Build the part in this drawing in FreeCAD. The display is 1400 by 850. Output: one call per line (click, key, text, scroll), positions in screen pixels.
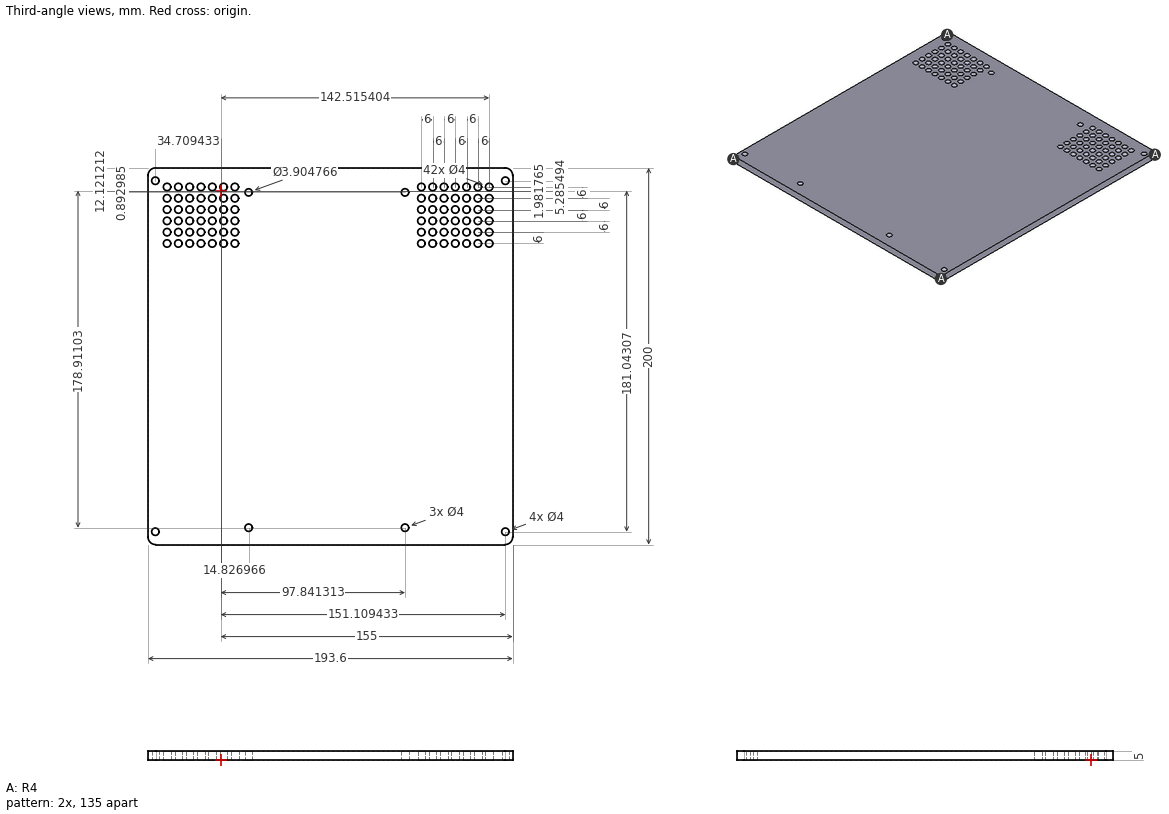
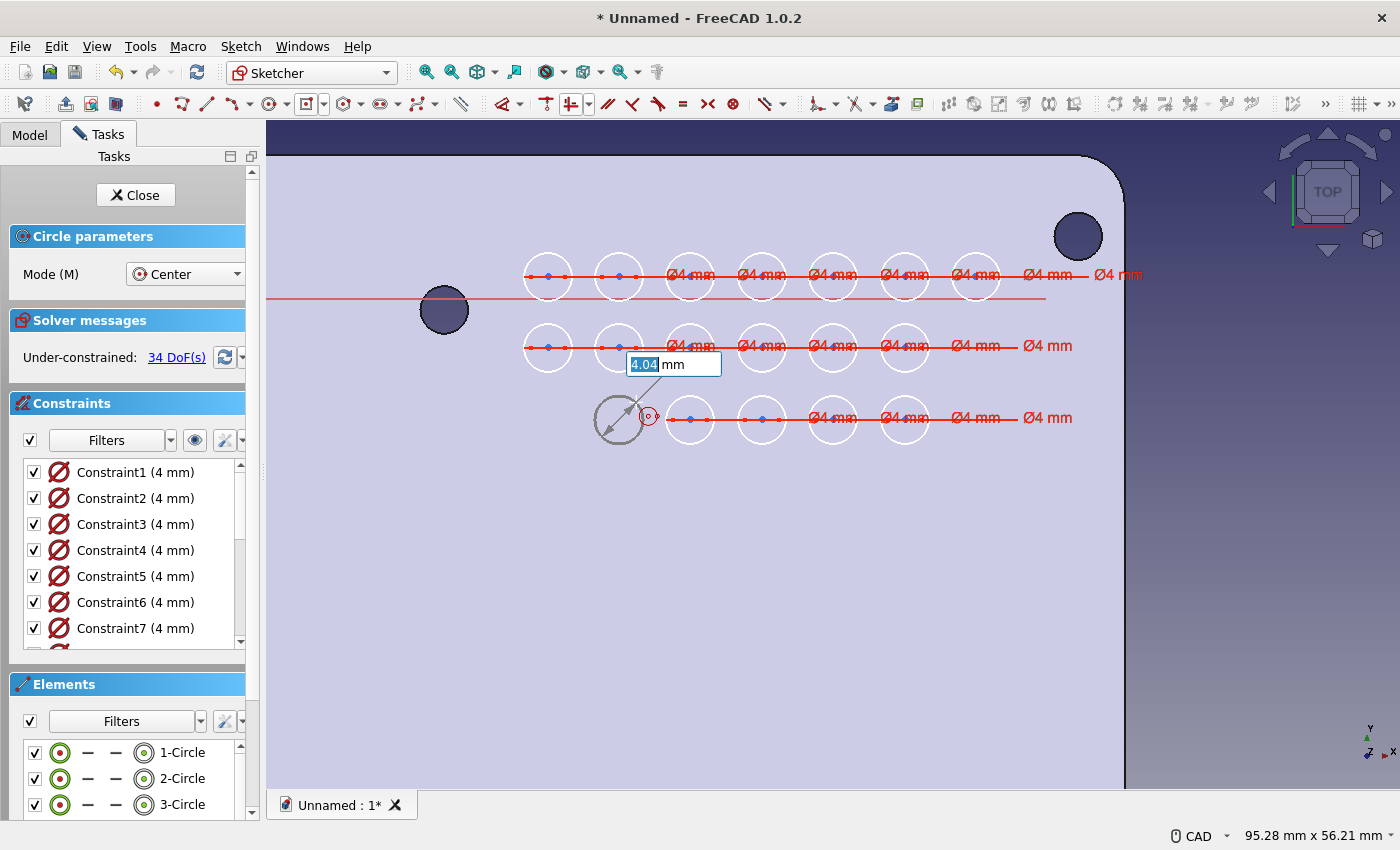
text(4)
key(Return)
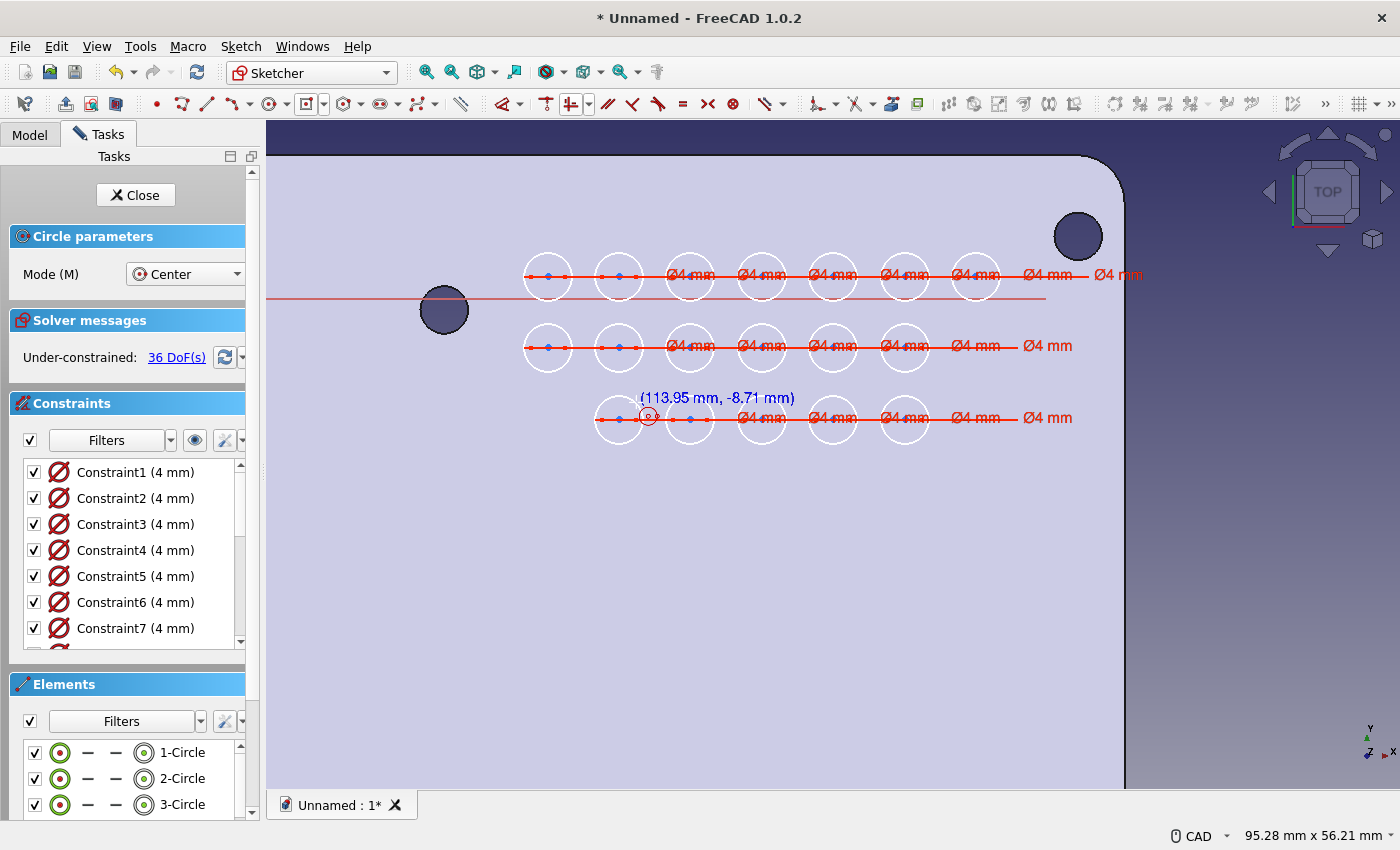
click(548, 419)
move(564, 402)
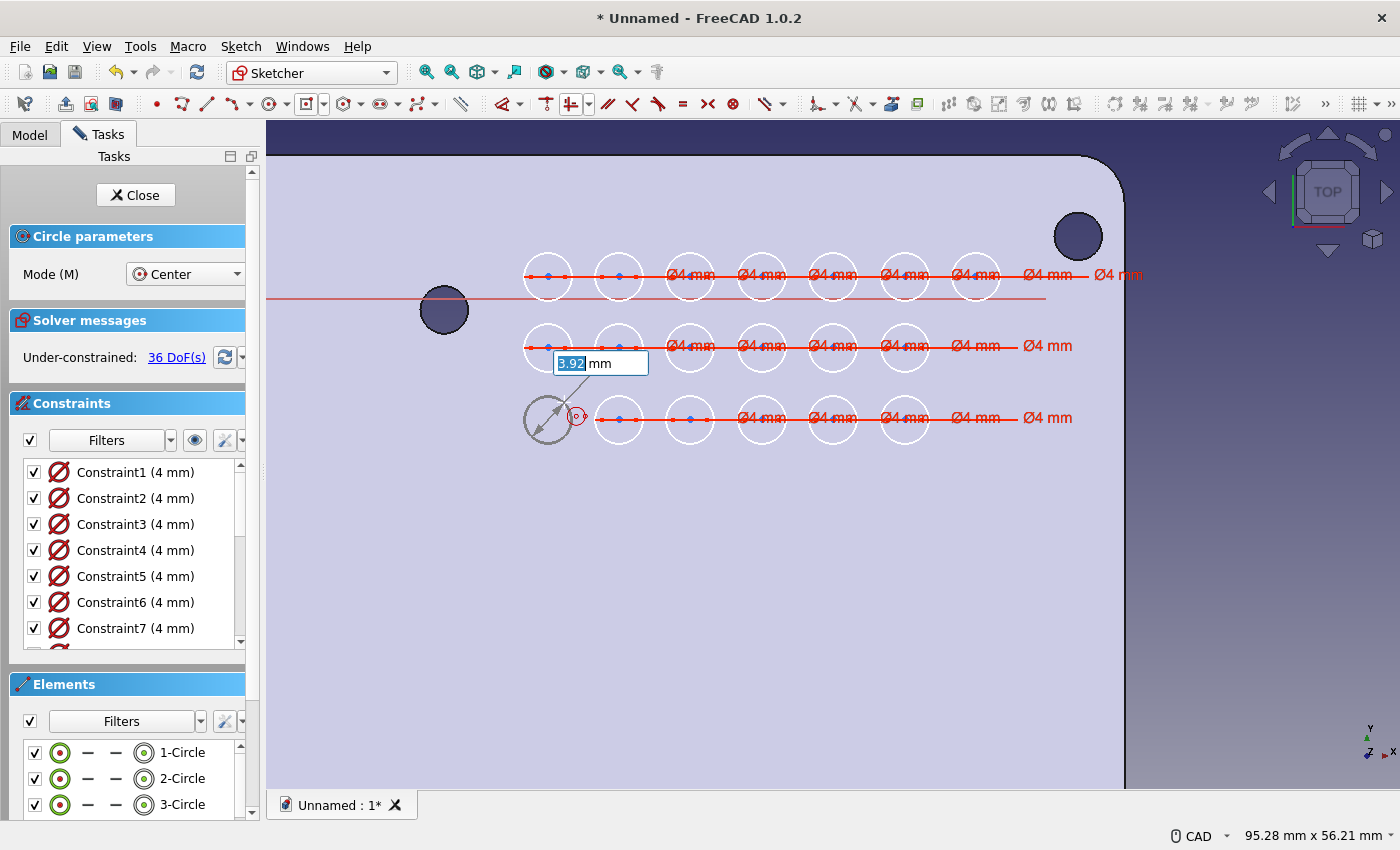
text(4)
key(Return)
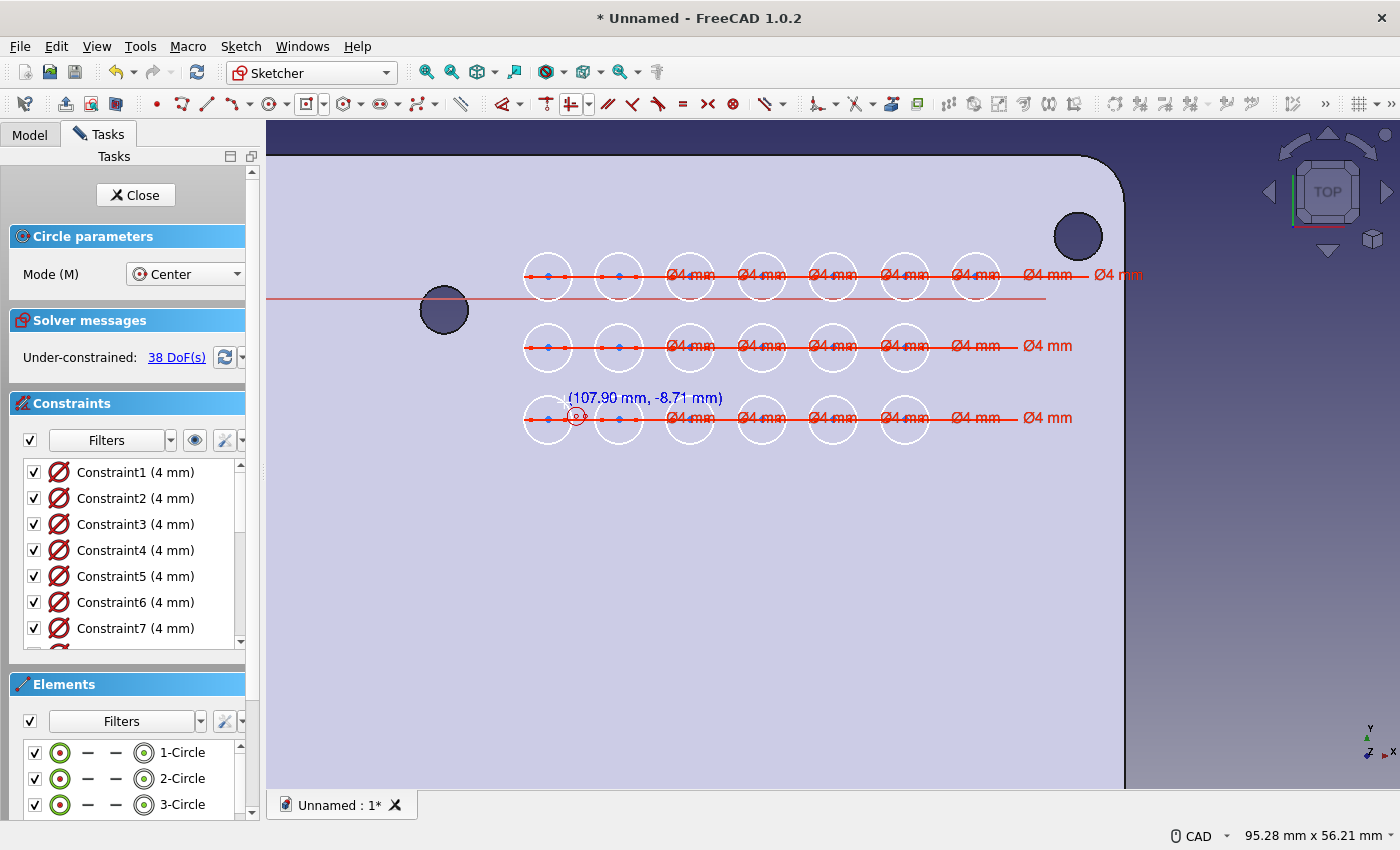
click(905, 490)
move(921, 473)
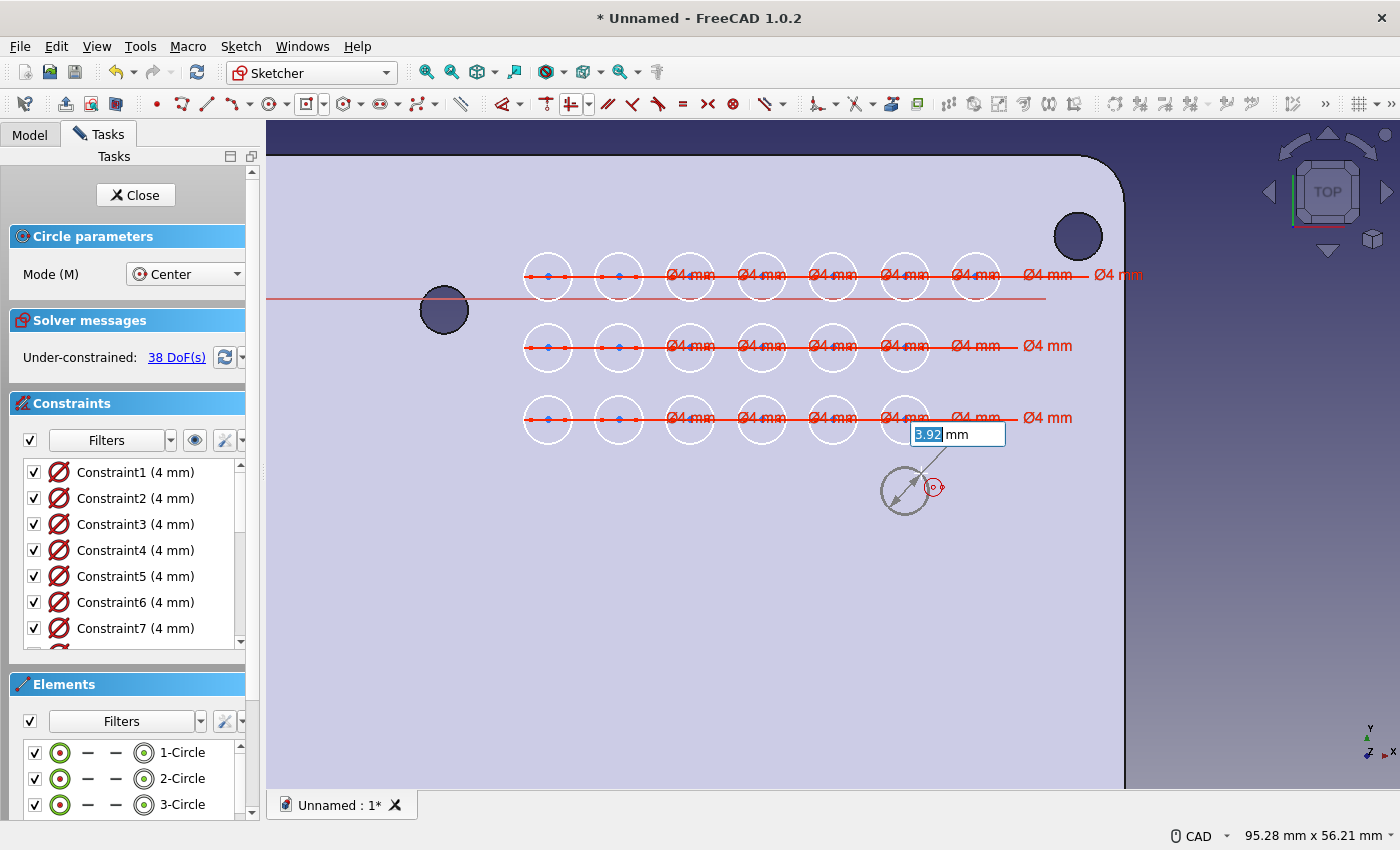
text(4)
key(Return)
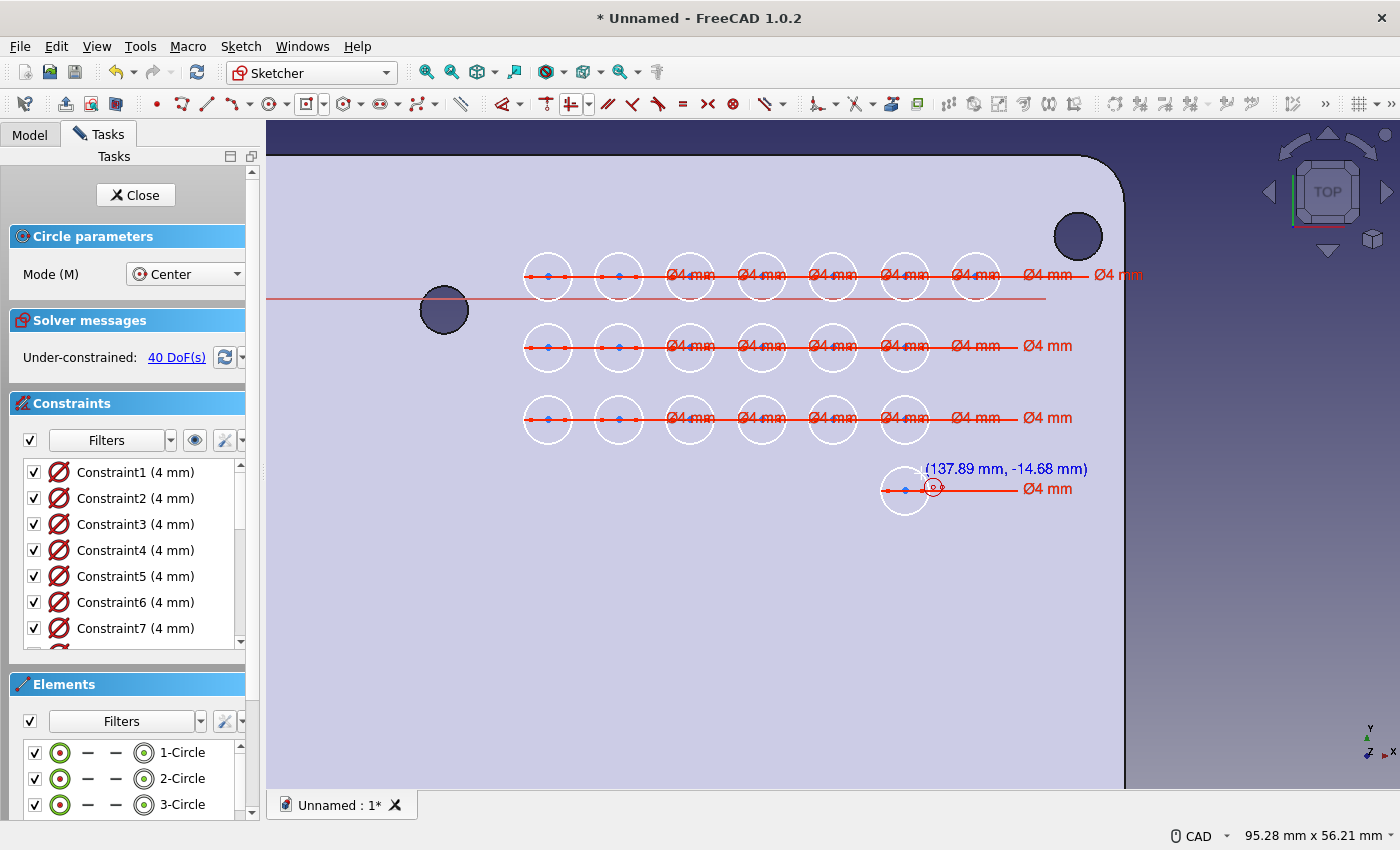
click(833, 490)
move(850, 473)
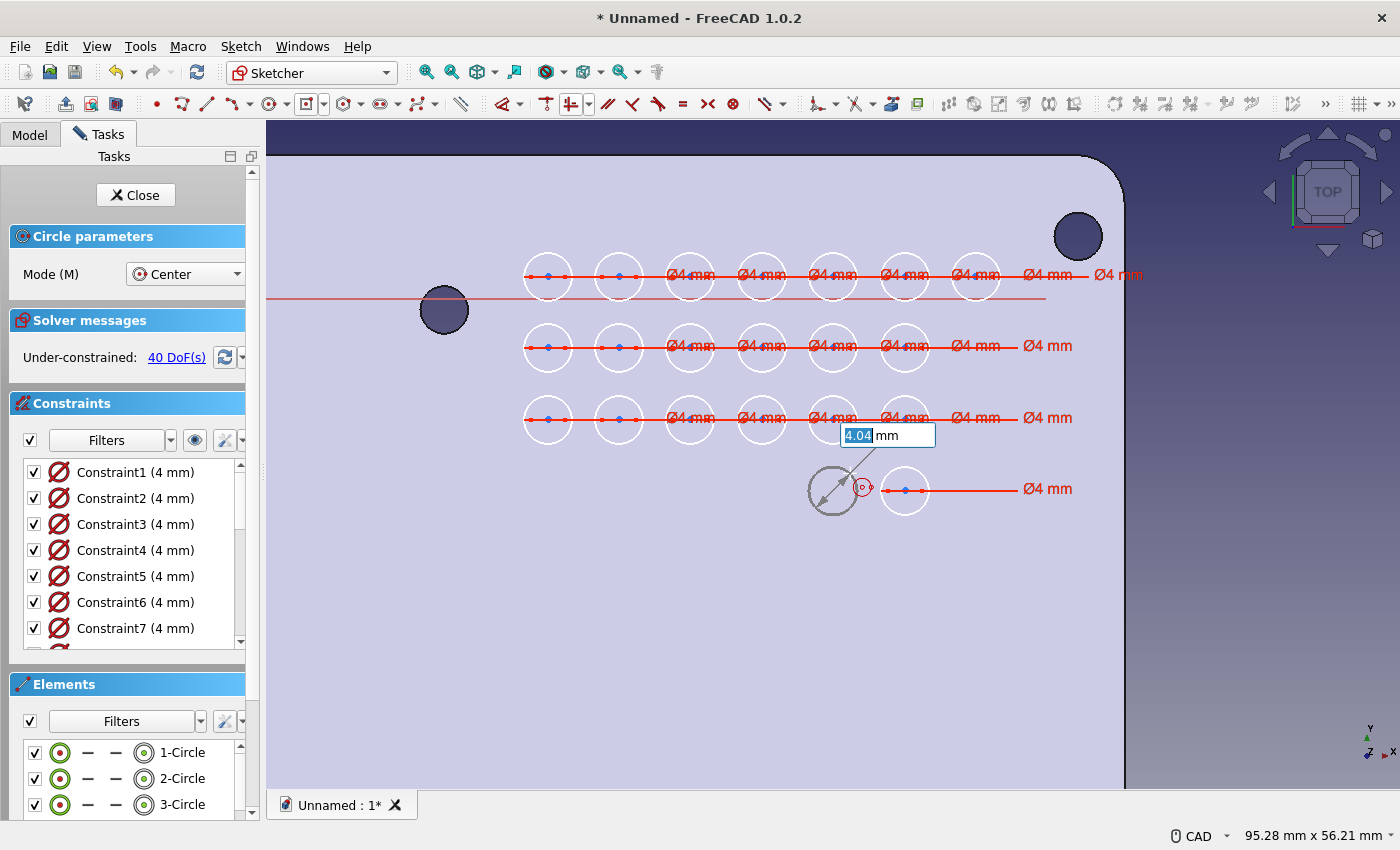
text(4)
key(Return)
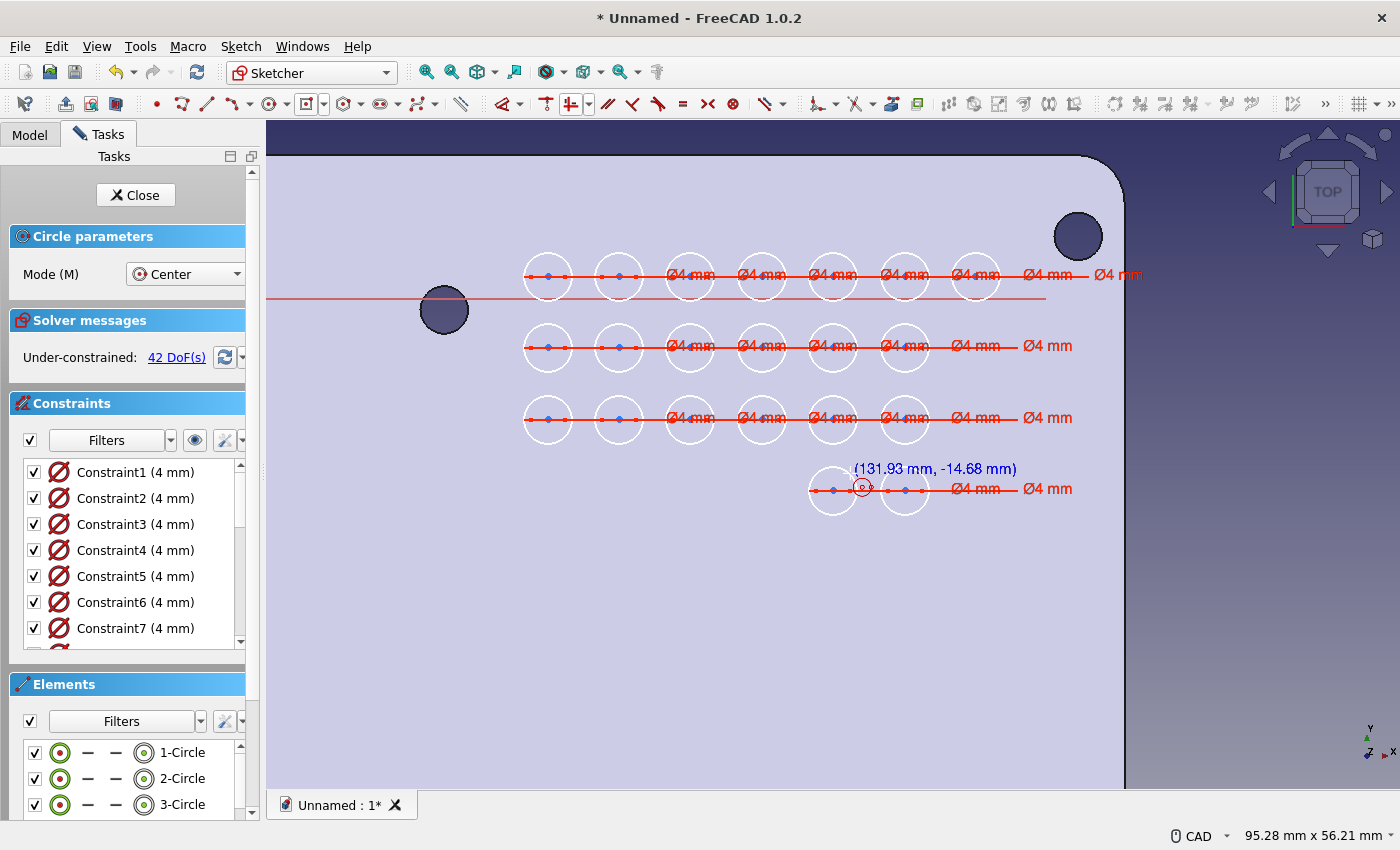
click(762, 490)
move(779, 473)